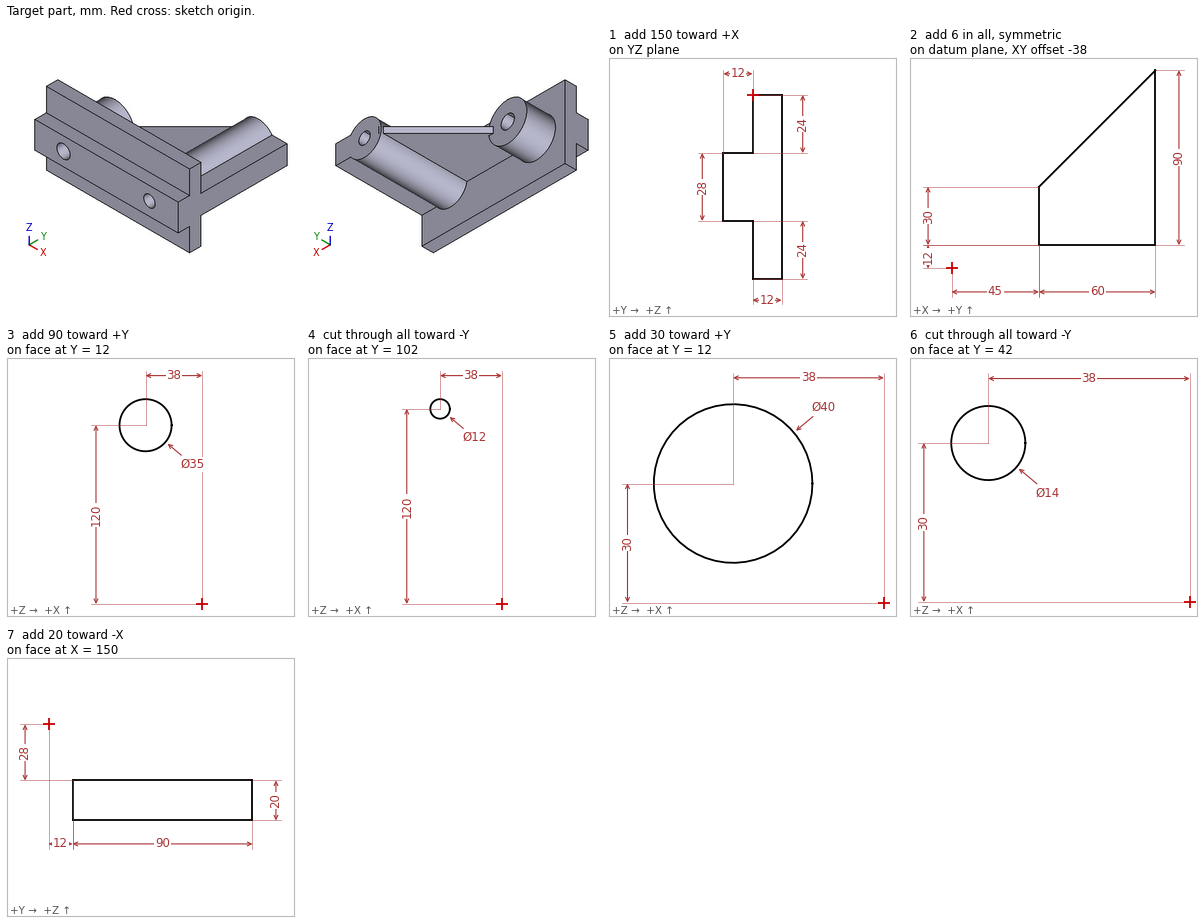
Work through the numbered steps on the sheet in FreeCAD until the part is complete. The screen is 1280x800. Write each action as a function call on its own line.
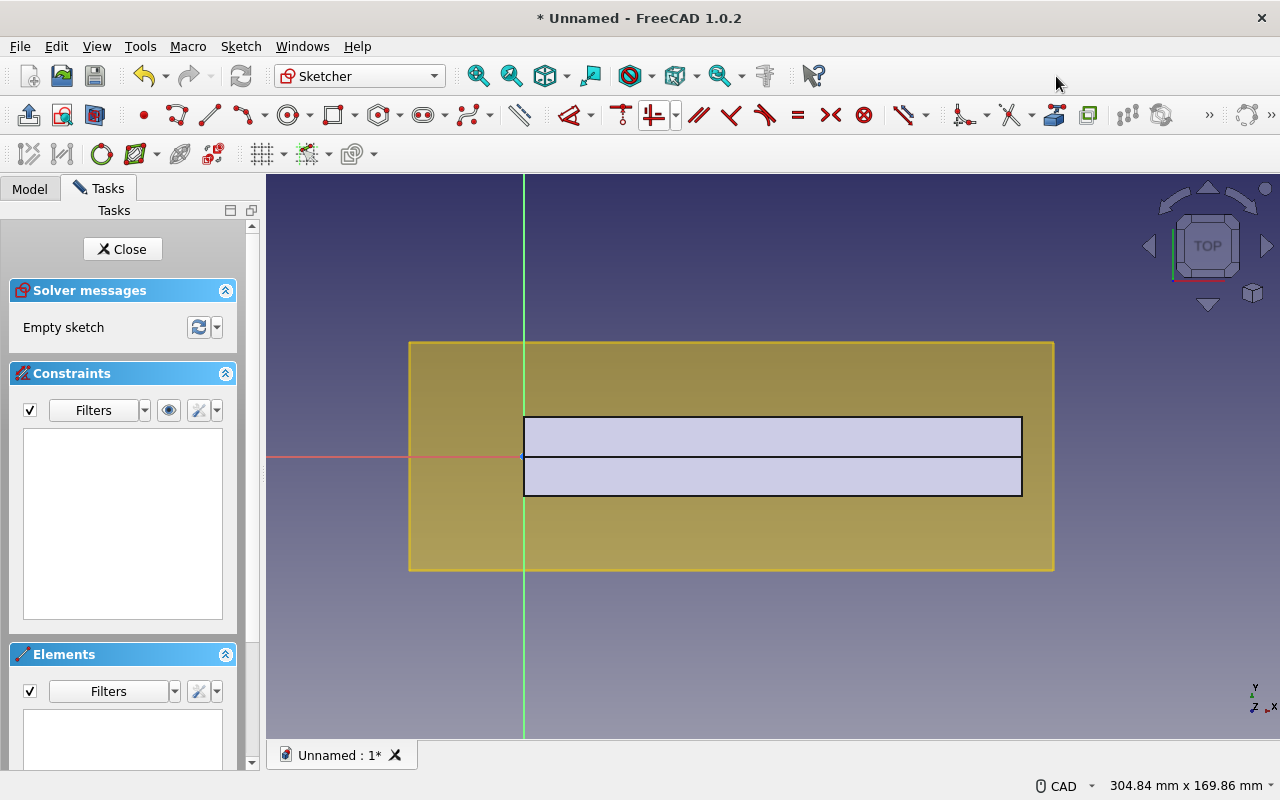
click(95, 116)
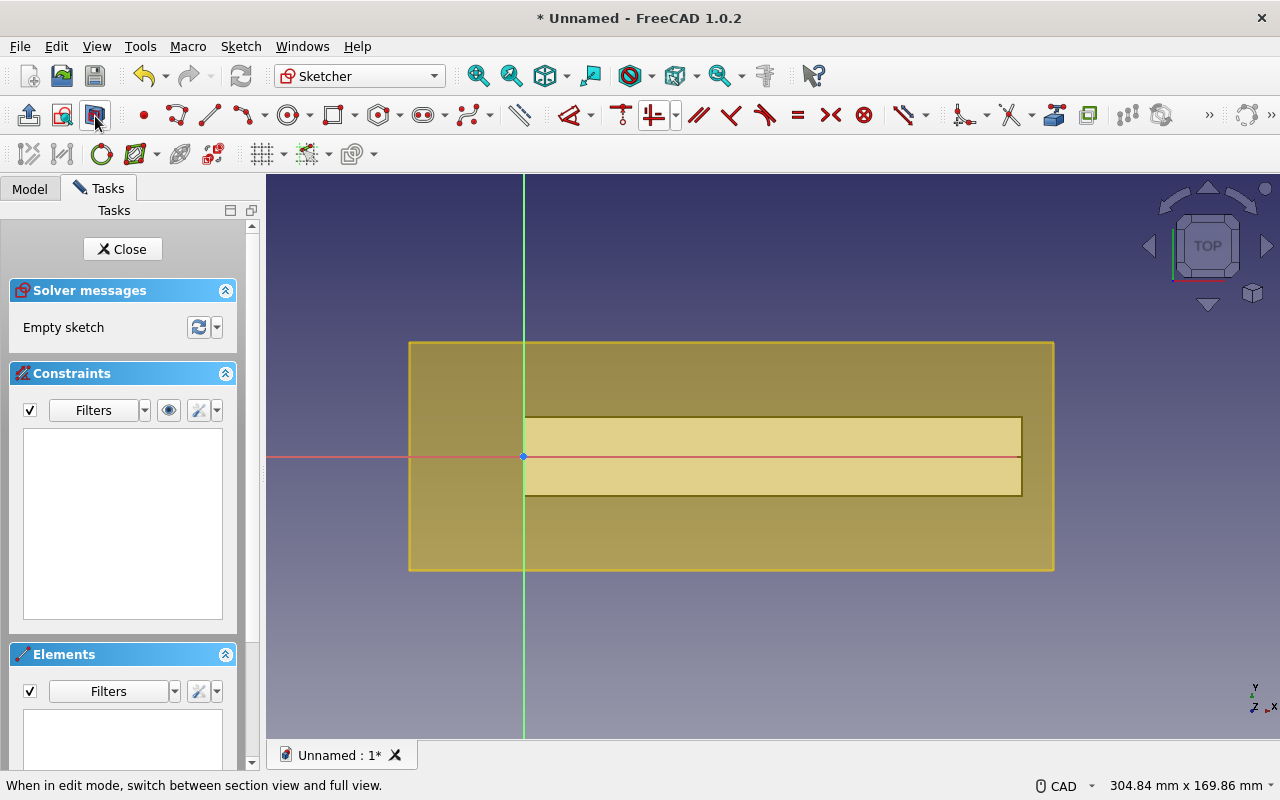
scroll(717, 711, down, 2)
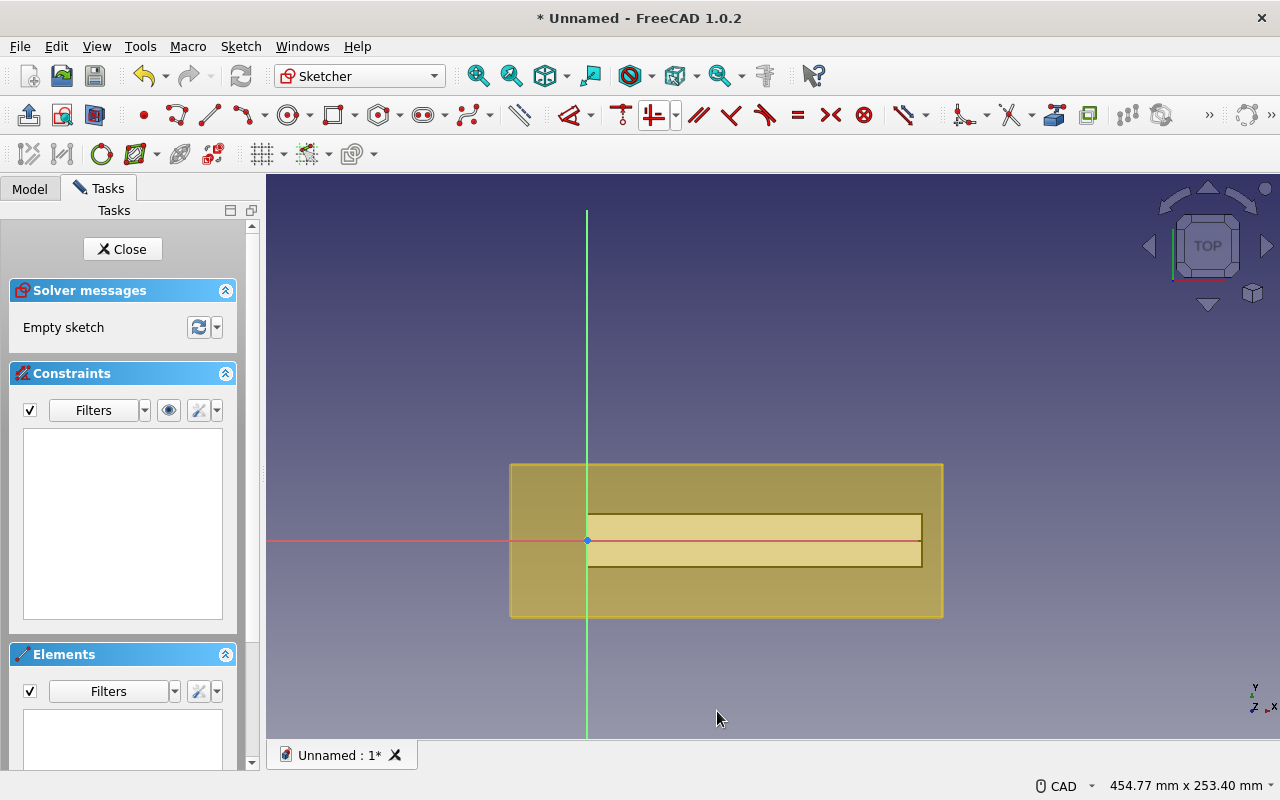
scroll(705, 367, up, 2)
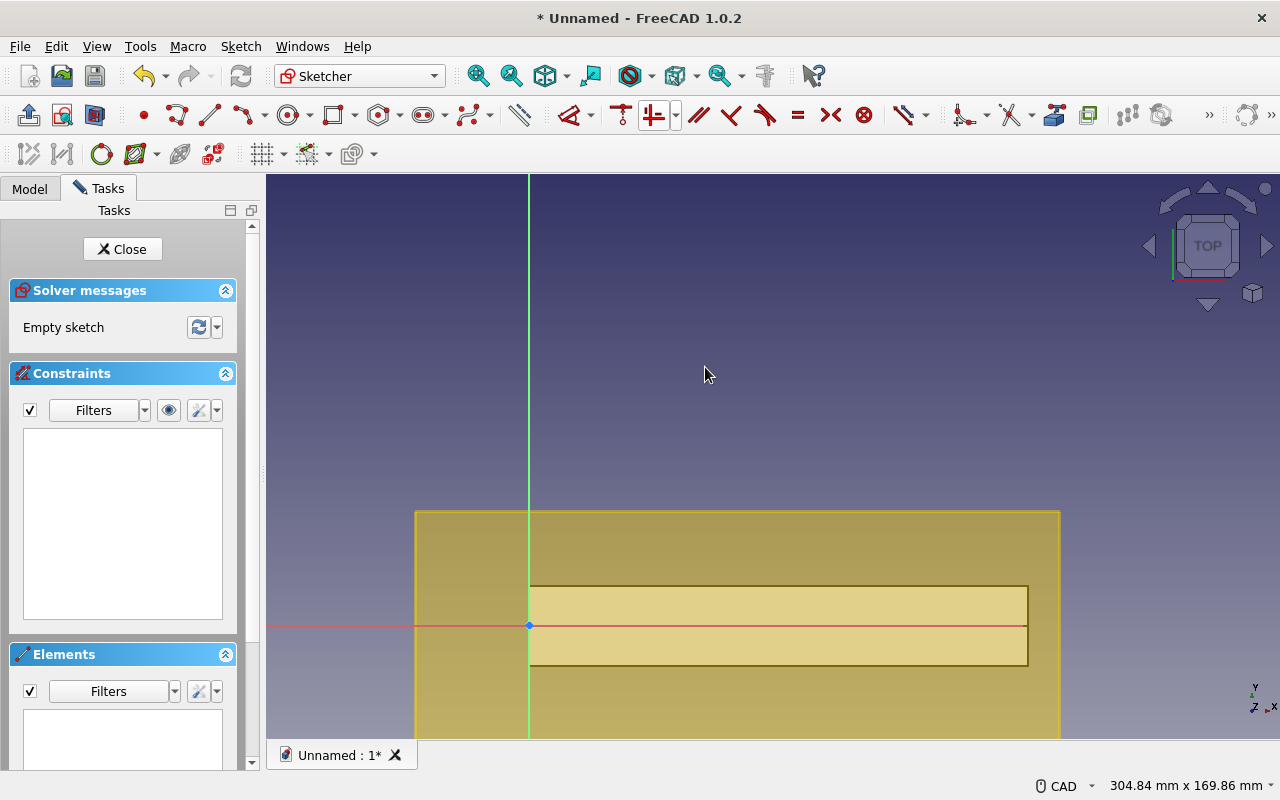
click(177, 116)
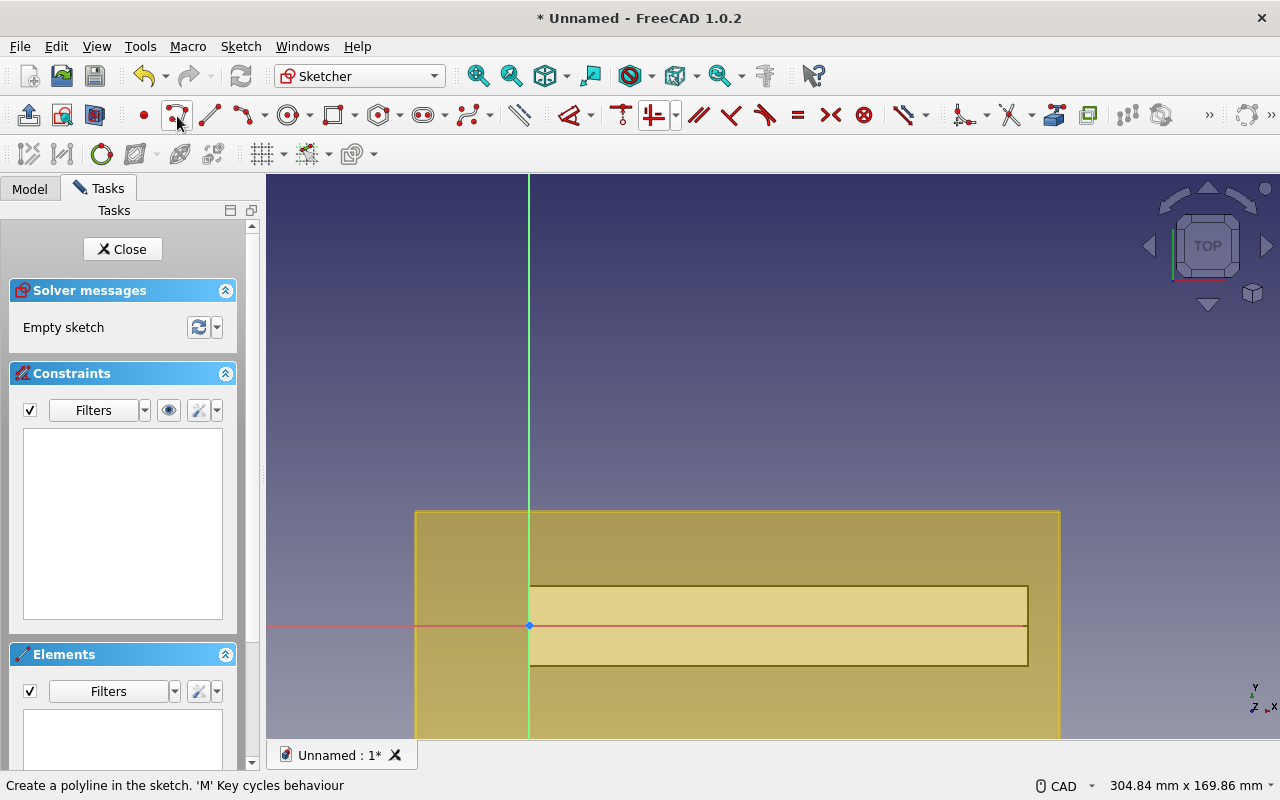
click(679, 586)
click(879, 586)
click(879, 287)
click(679, 486)
click(679, 587)
key(Escape)
key(Escape)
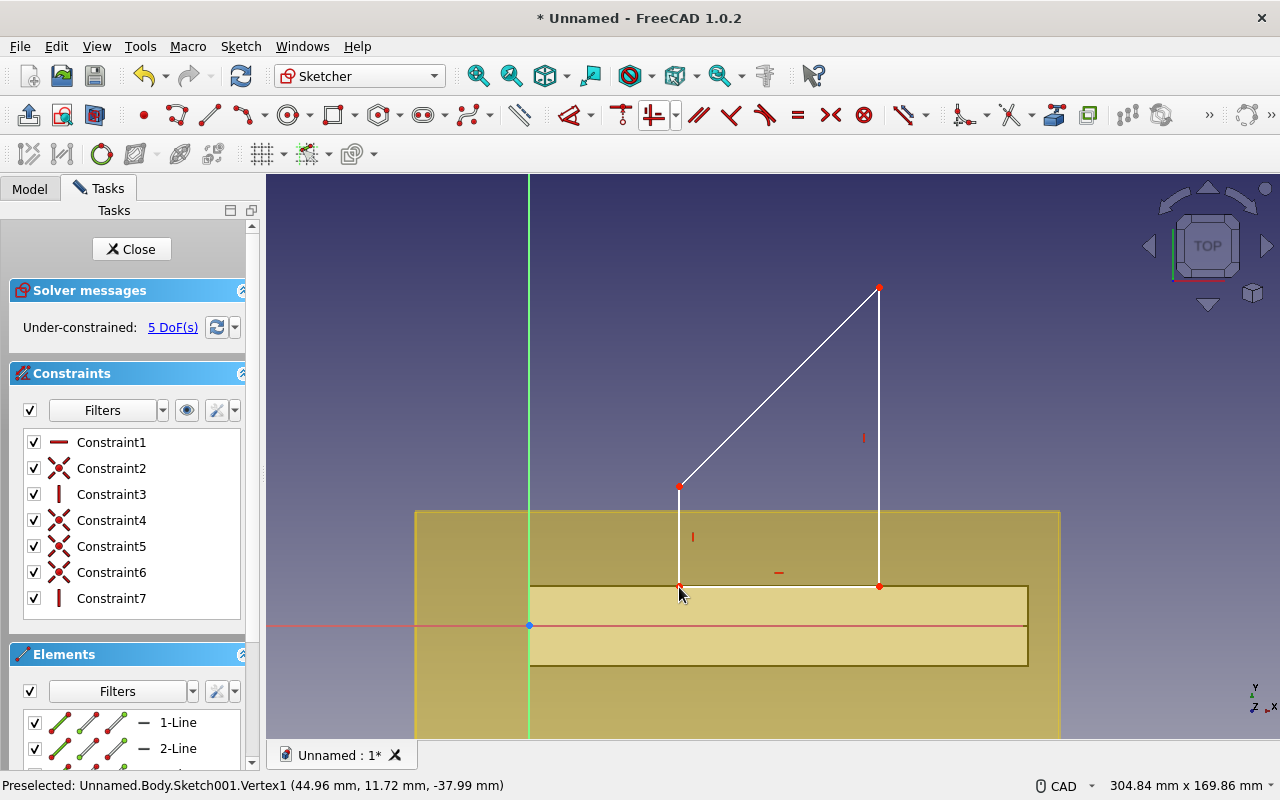
click(568, 116)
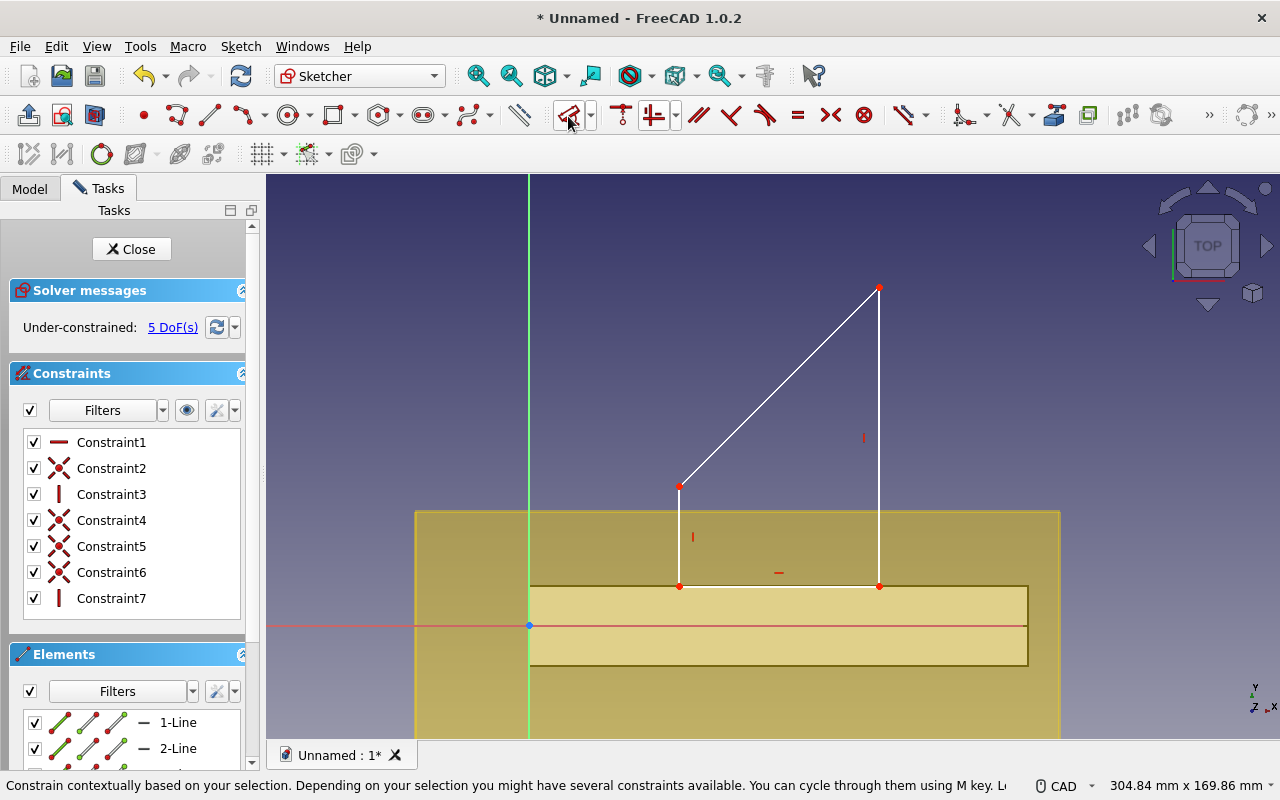
click(739, 587)
click(779, 553)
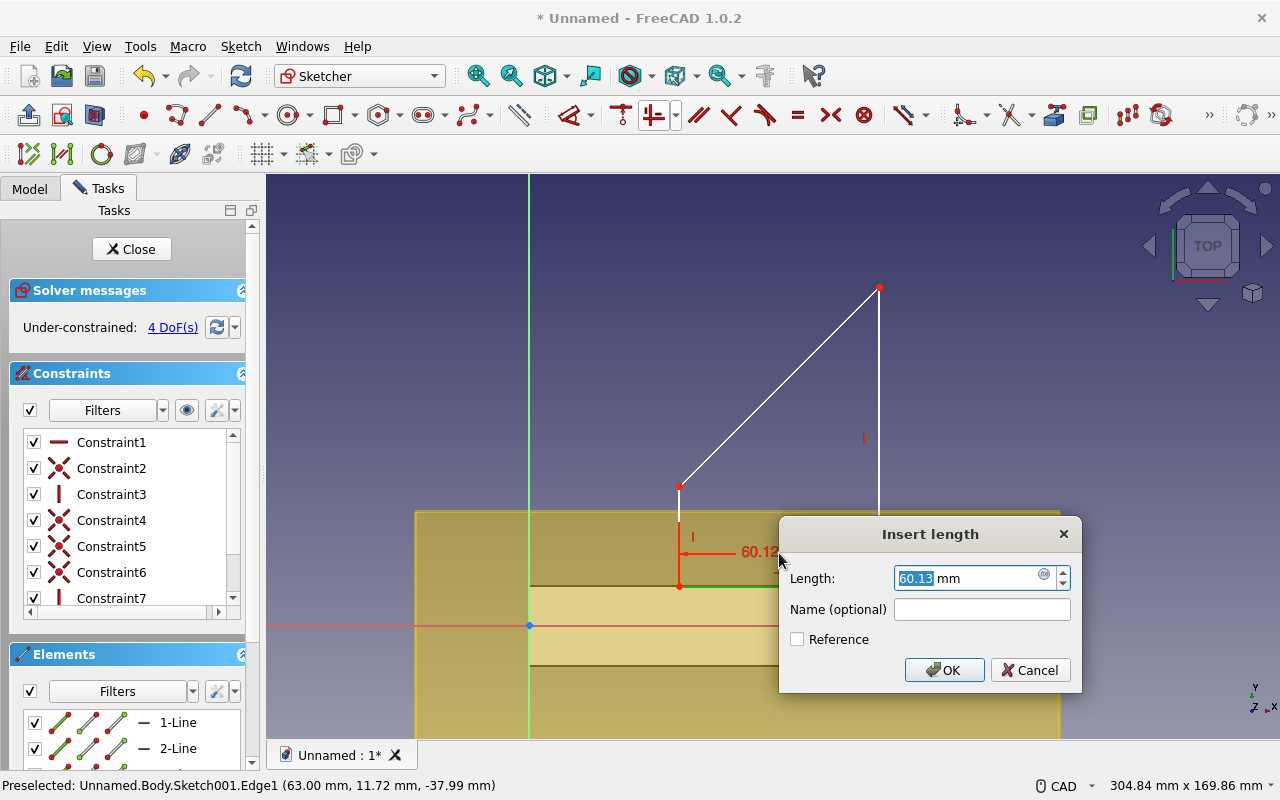
text(60)
key(Return)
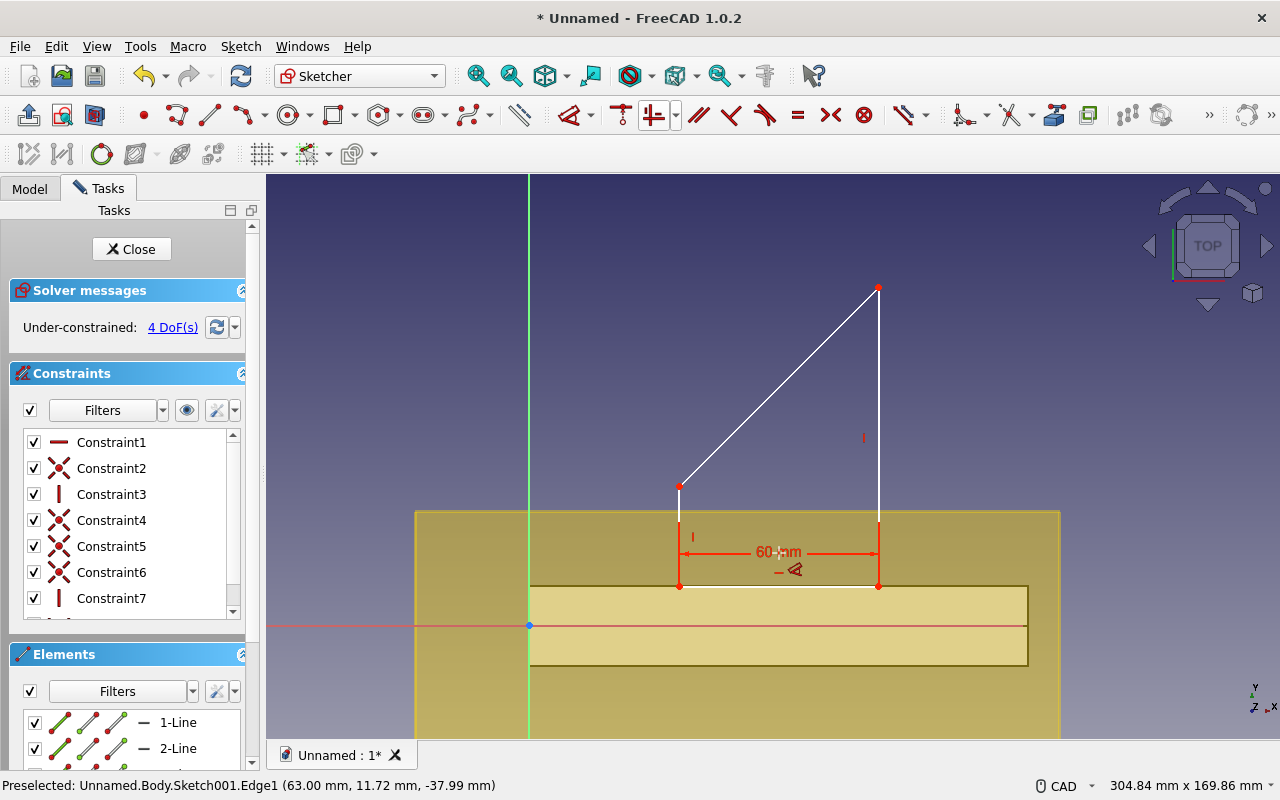
click(879, 497)
click(913, 437)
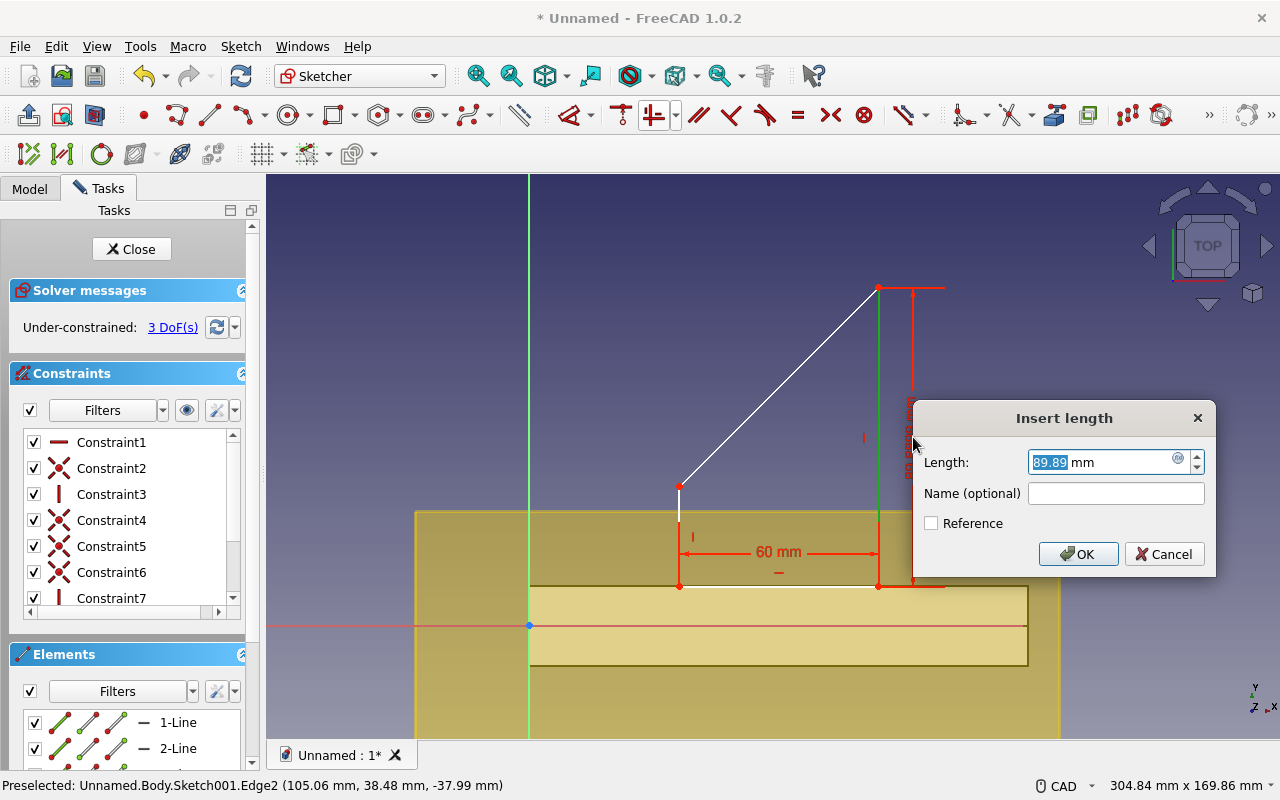
text(90)
key(Return)